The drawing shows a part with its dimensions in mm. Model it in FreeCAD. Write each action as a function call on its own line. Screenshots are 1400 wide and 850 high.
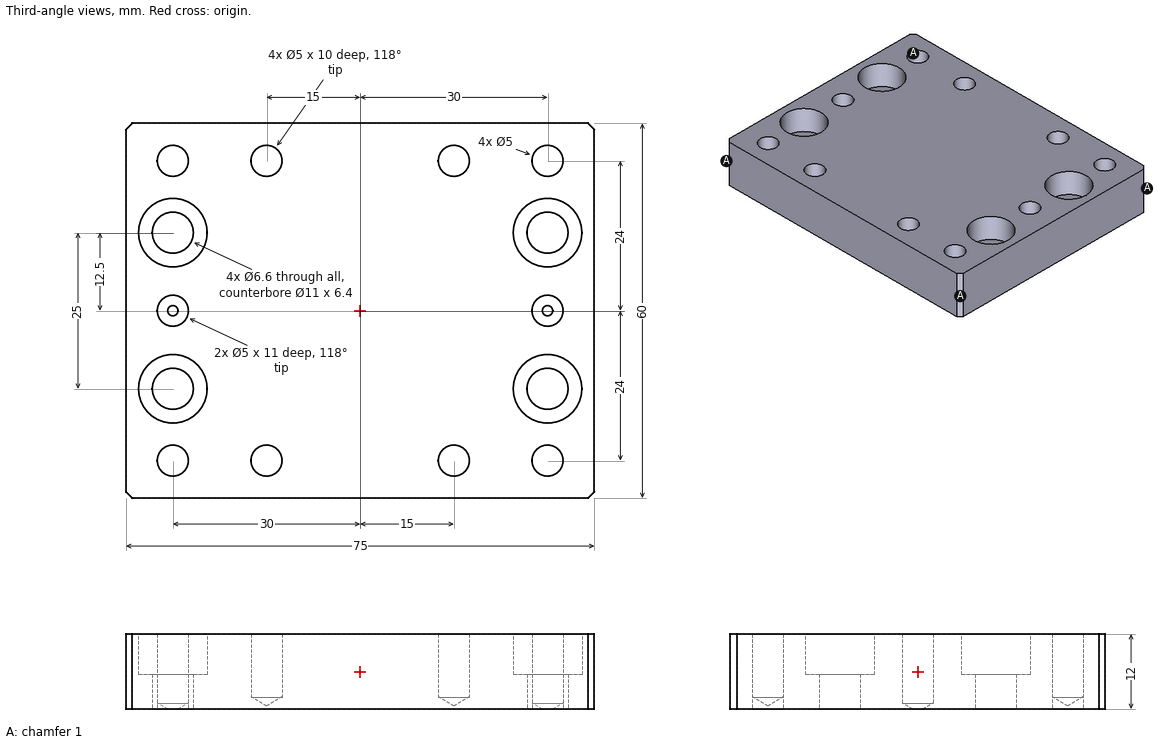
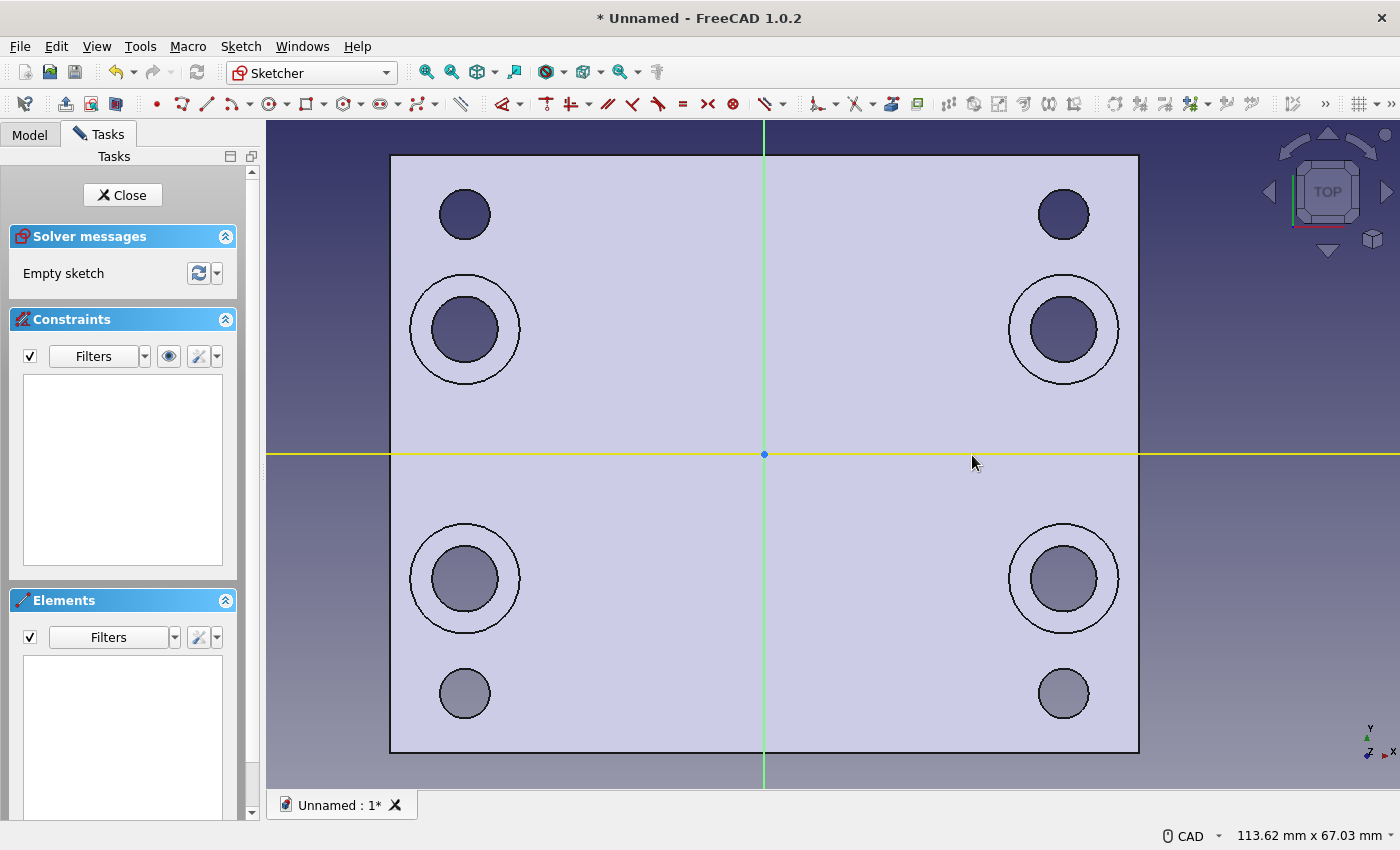
key(g)
key(c)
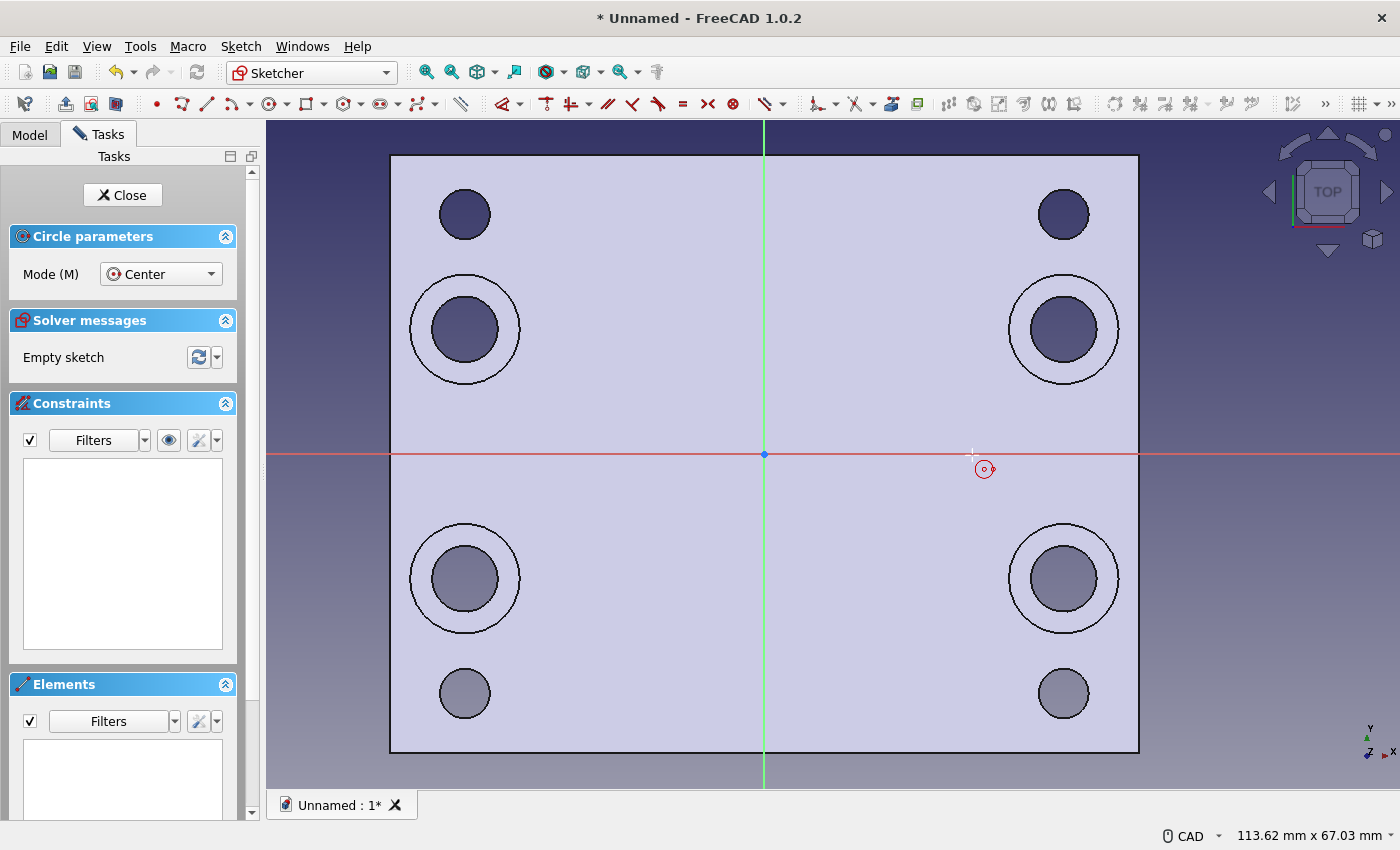
click(465, 454)
click(483, 436)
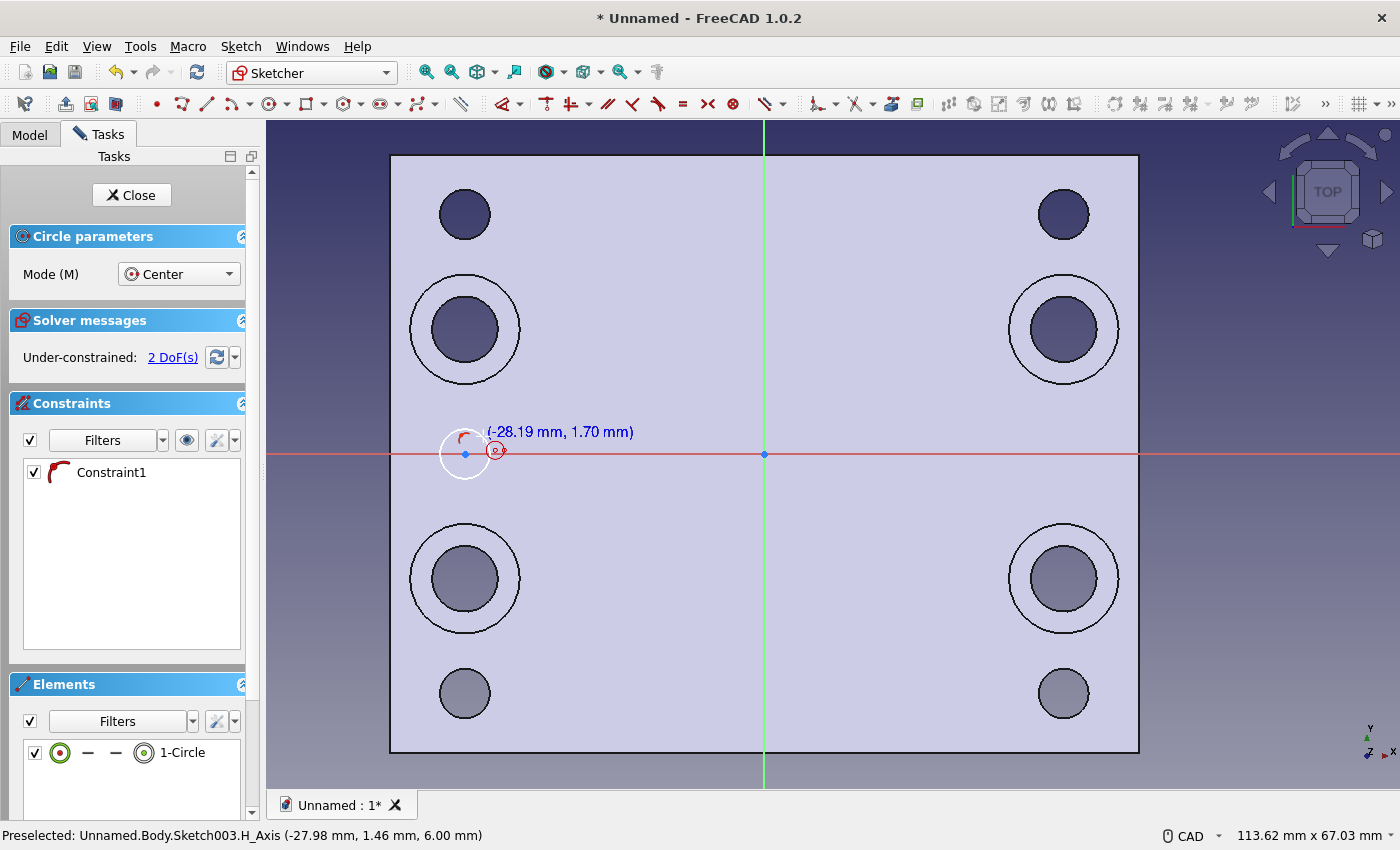
click(1064, 454)
click(1081, 436)
key(Escape)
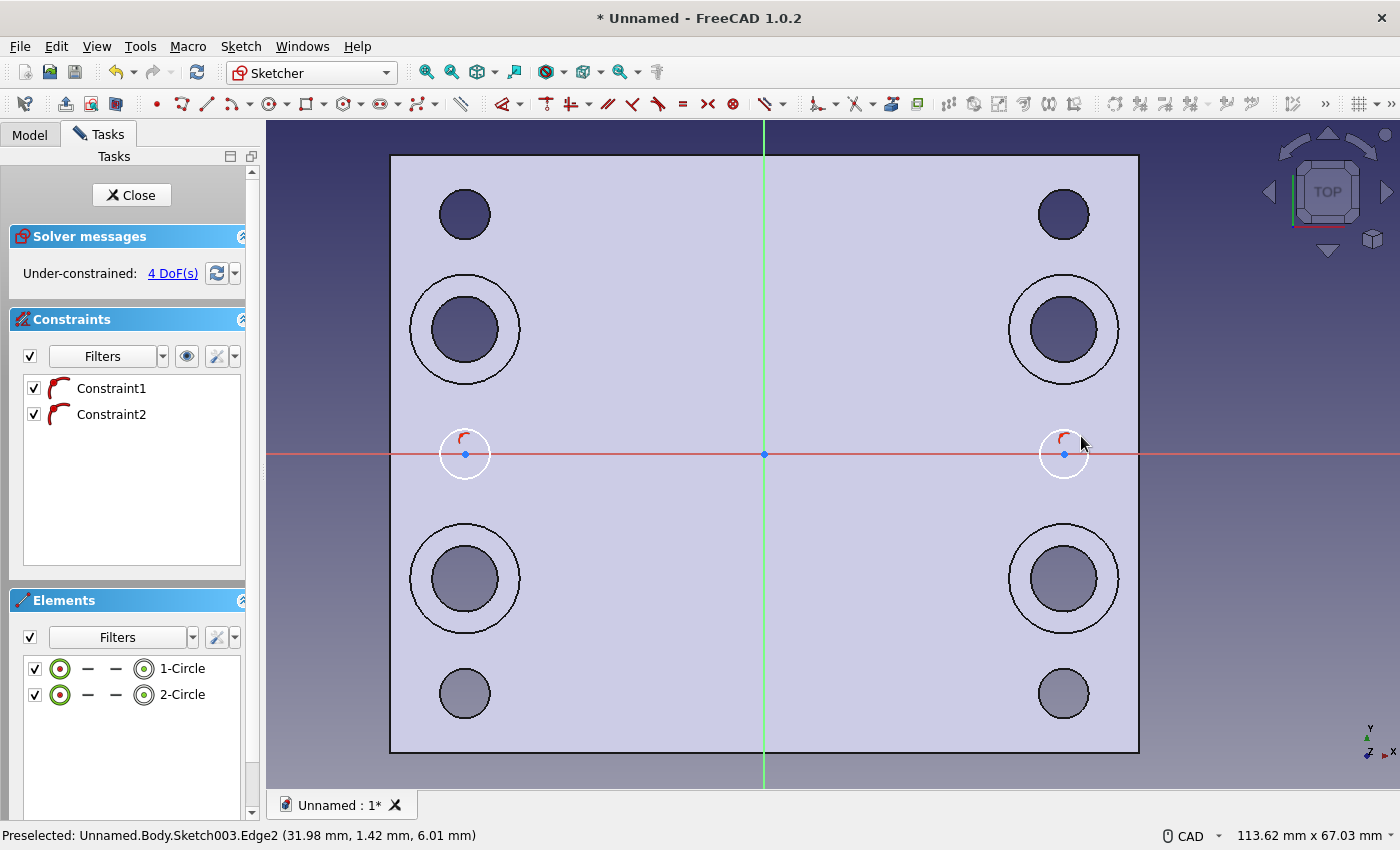
click(482, 436)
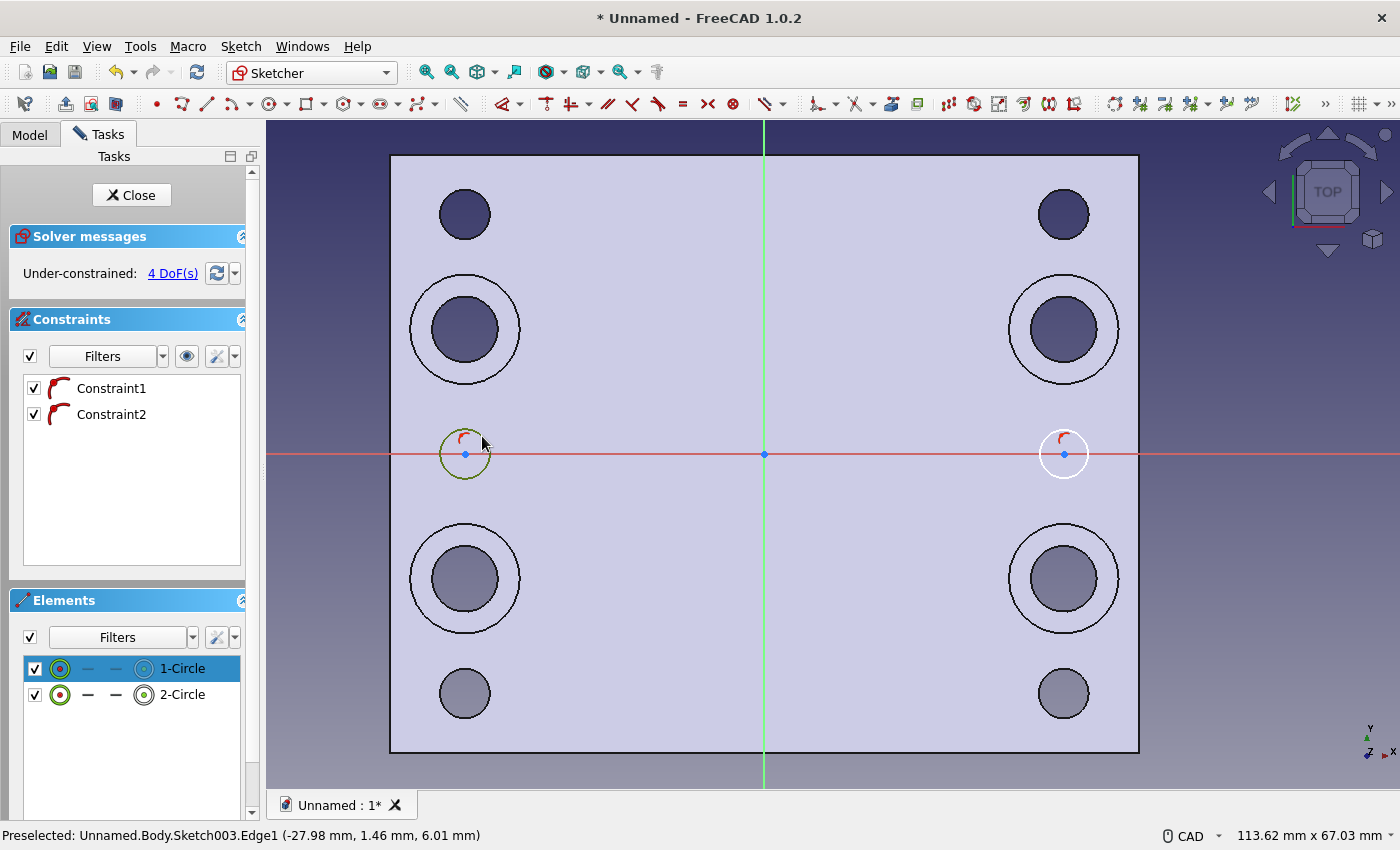
click(1081, 437)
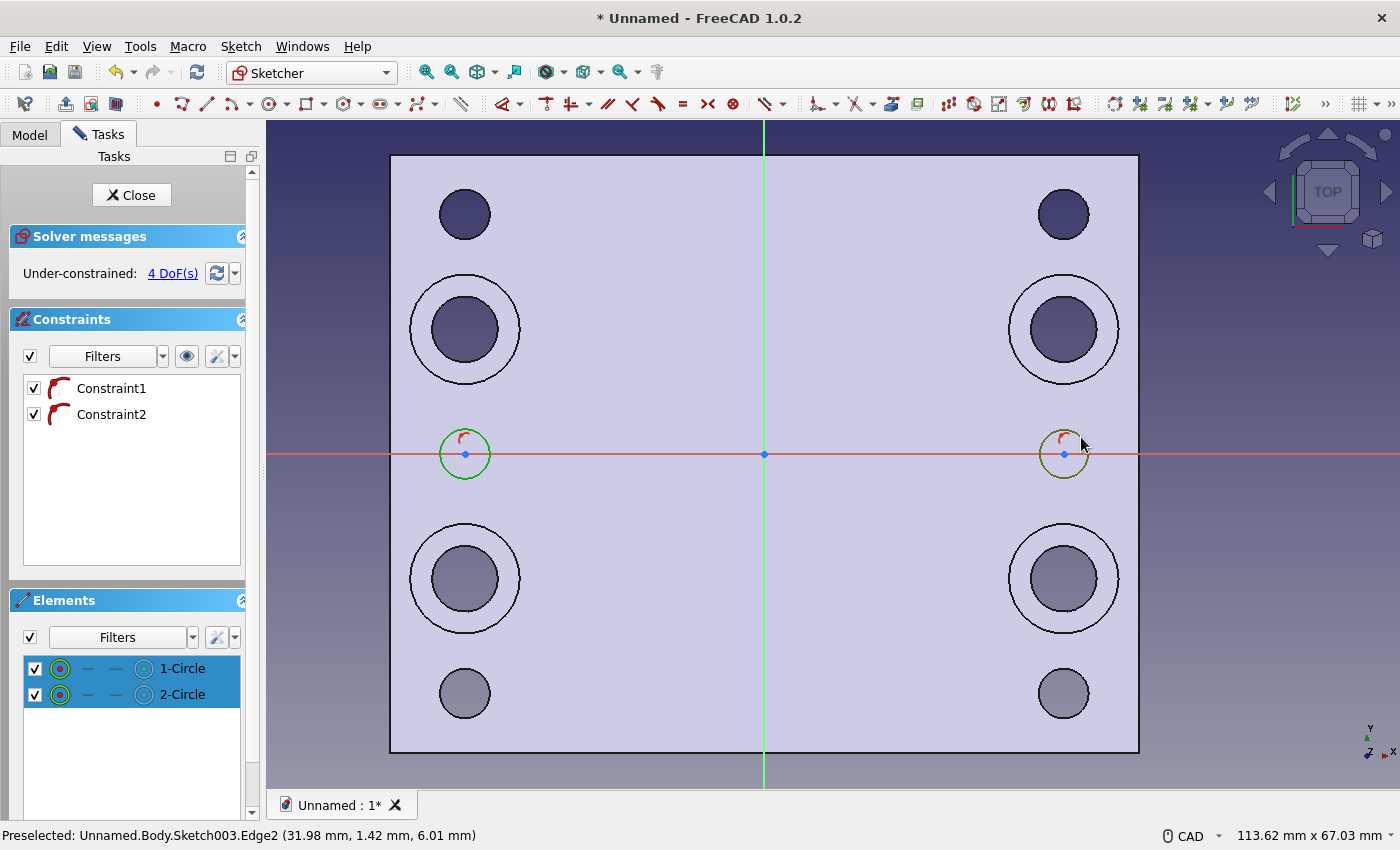
click(683, 104)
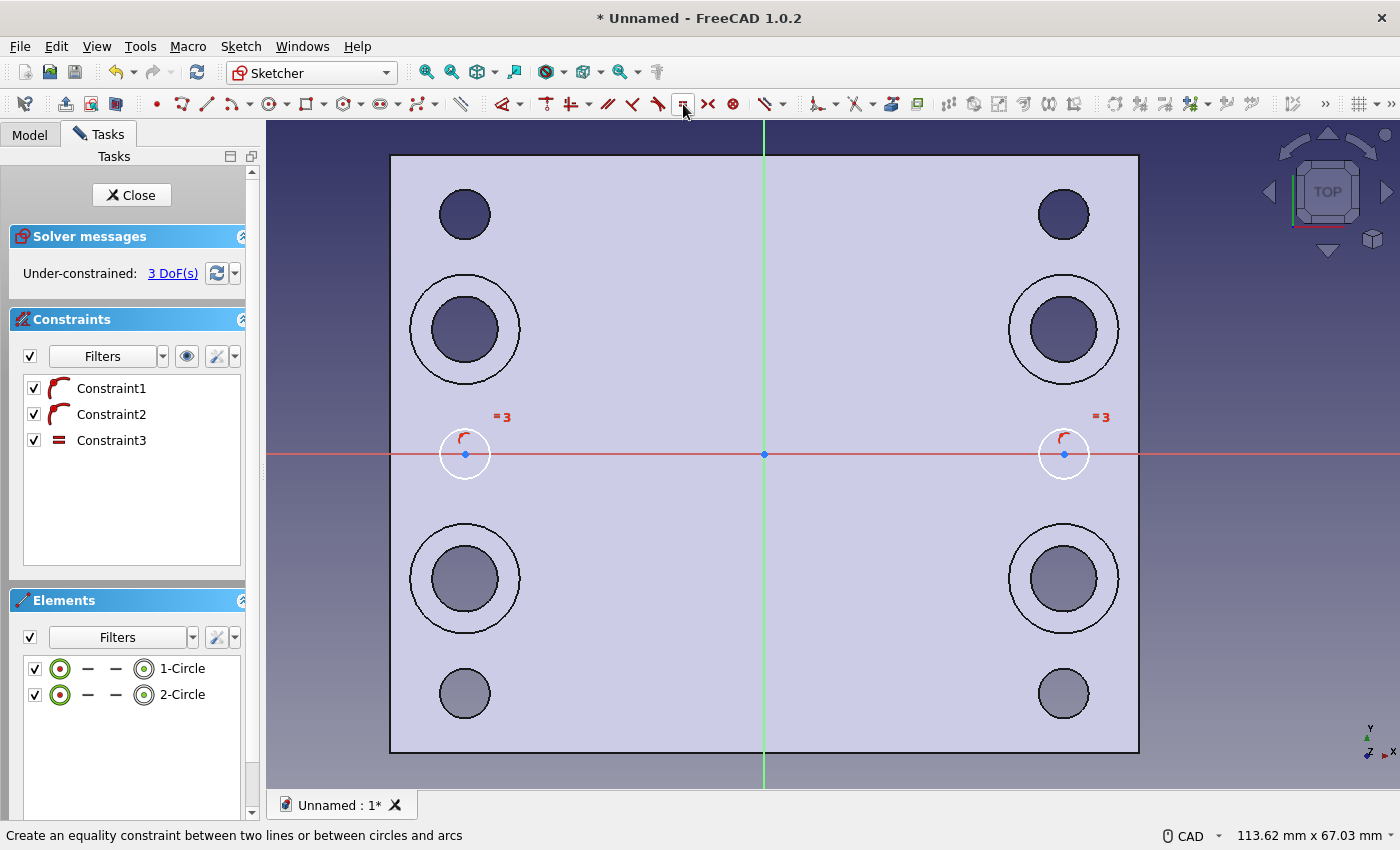
click(502, 104)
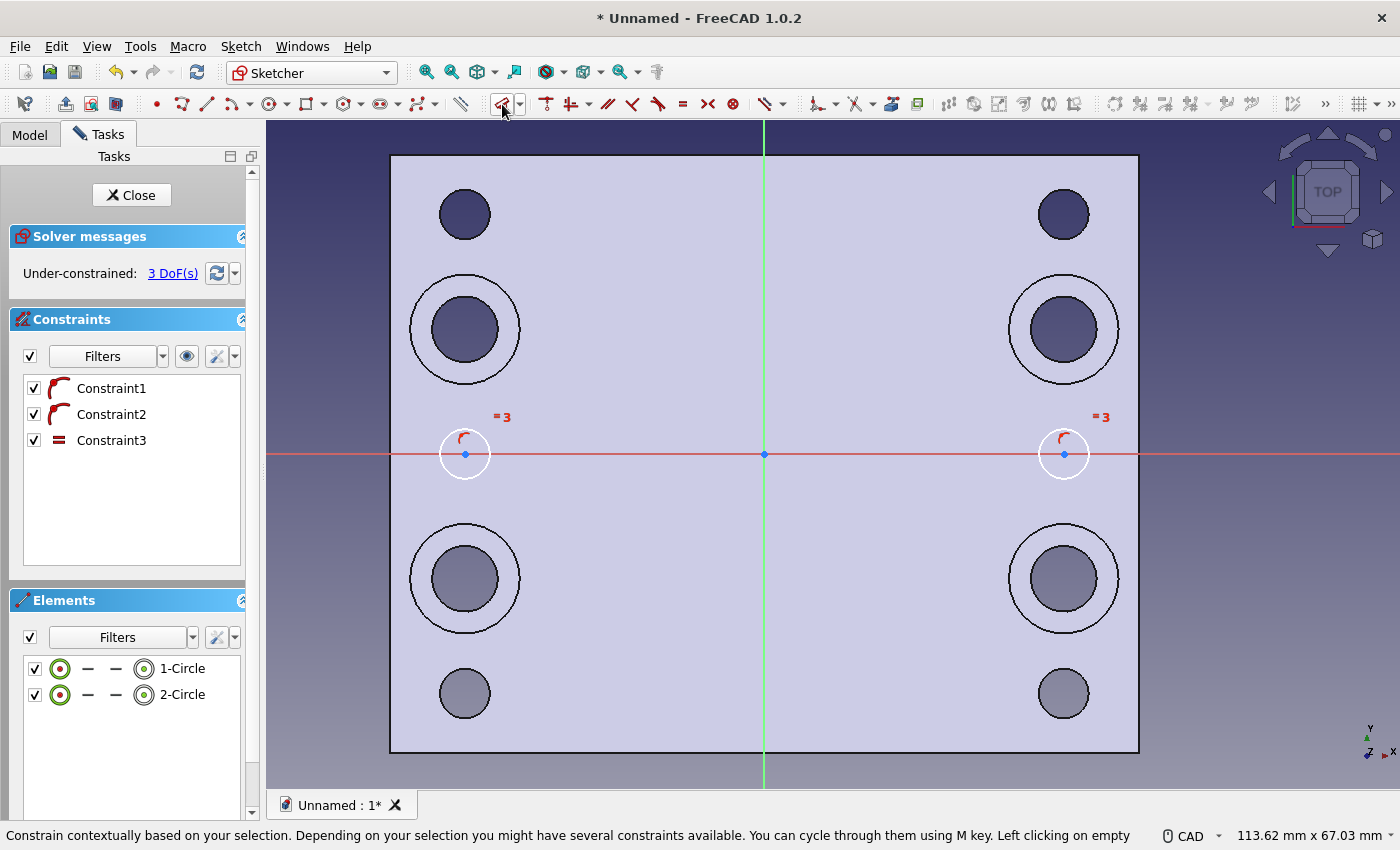
click(482, 436)
click(504, 413)